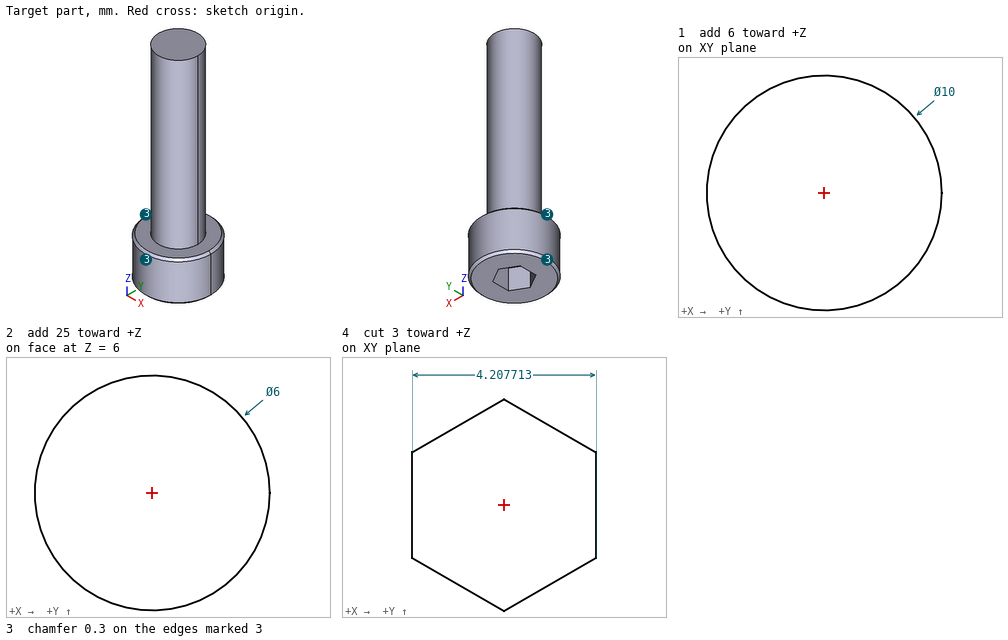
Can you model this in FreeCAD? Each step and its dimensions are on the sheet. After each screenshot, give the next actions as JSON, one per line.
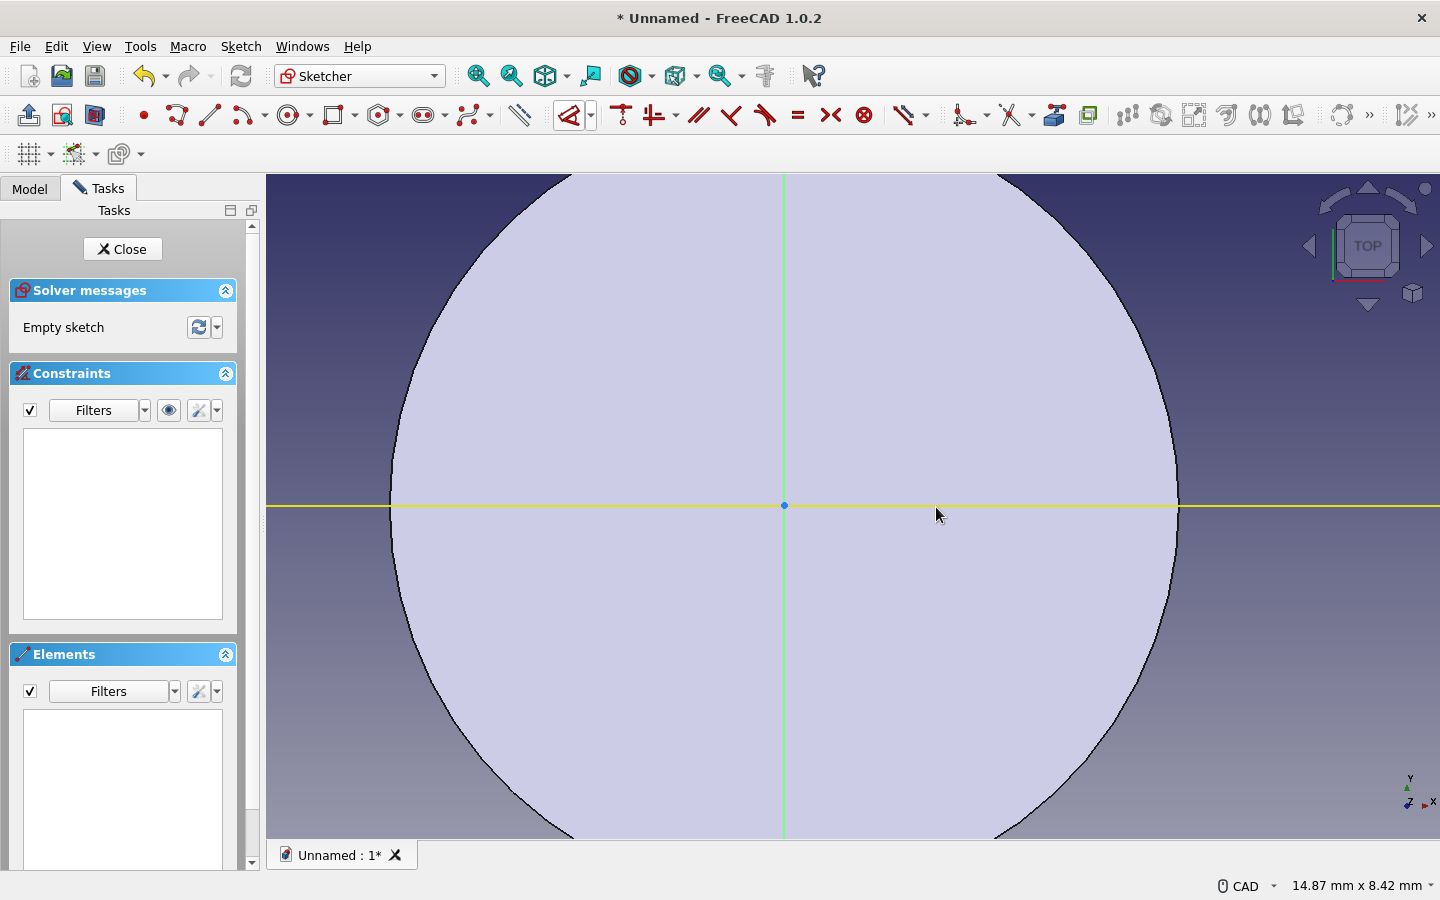
{"action": "left_click", "coordinate": [288, 116]}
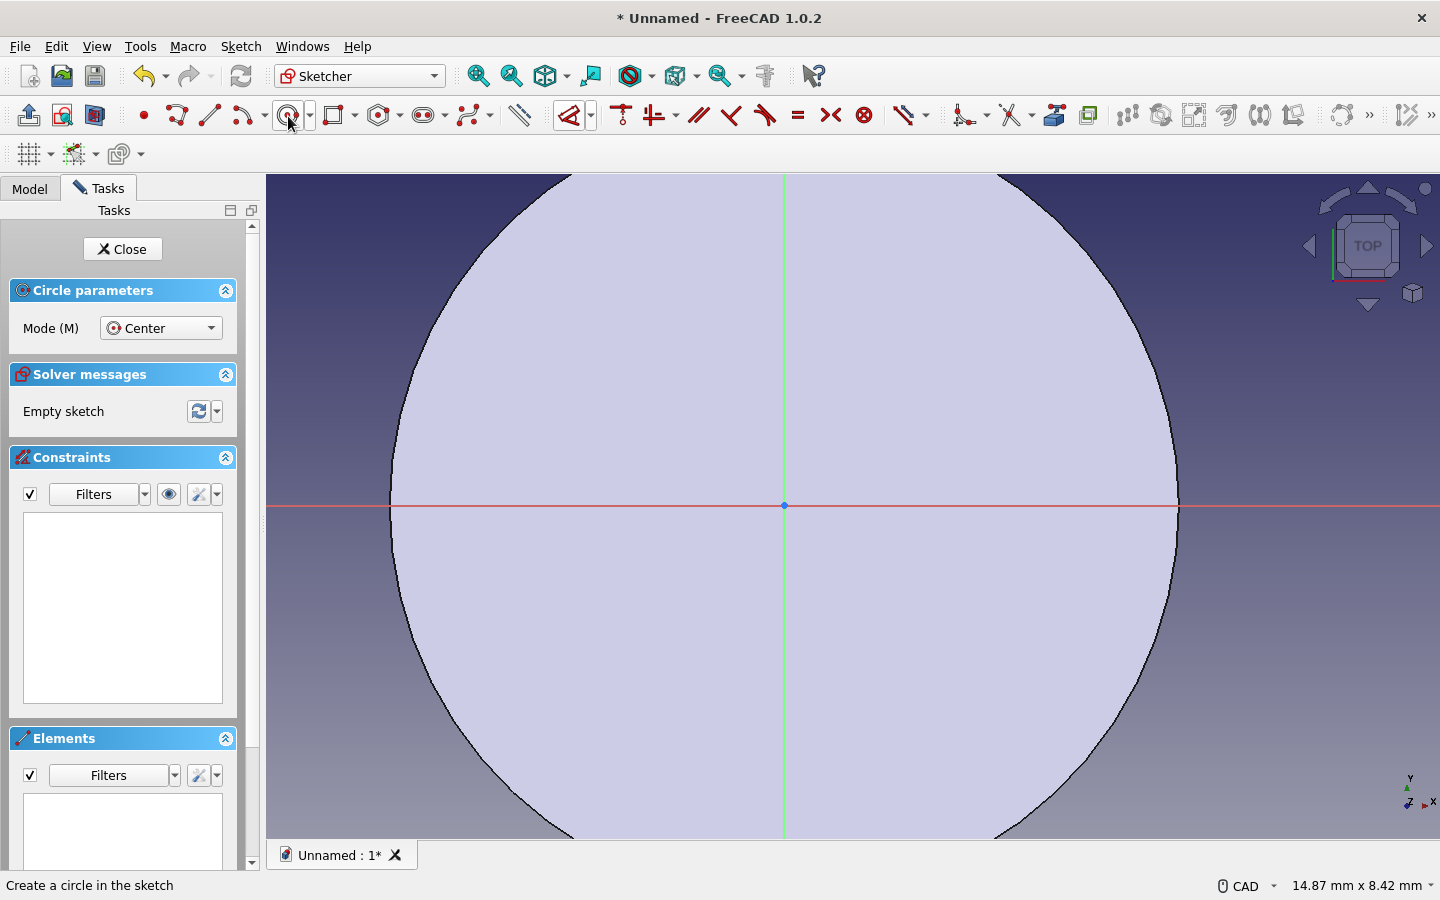
{"action": "left_click", "coordinate": [784, 506]}
{"action": "mouse_move", "coordinate": [952, 338]}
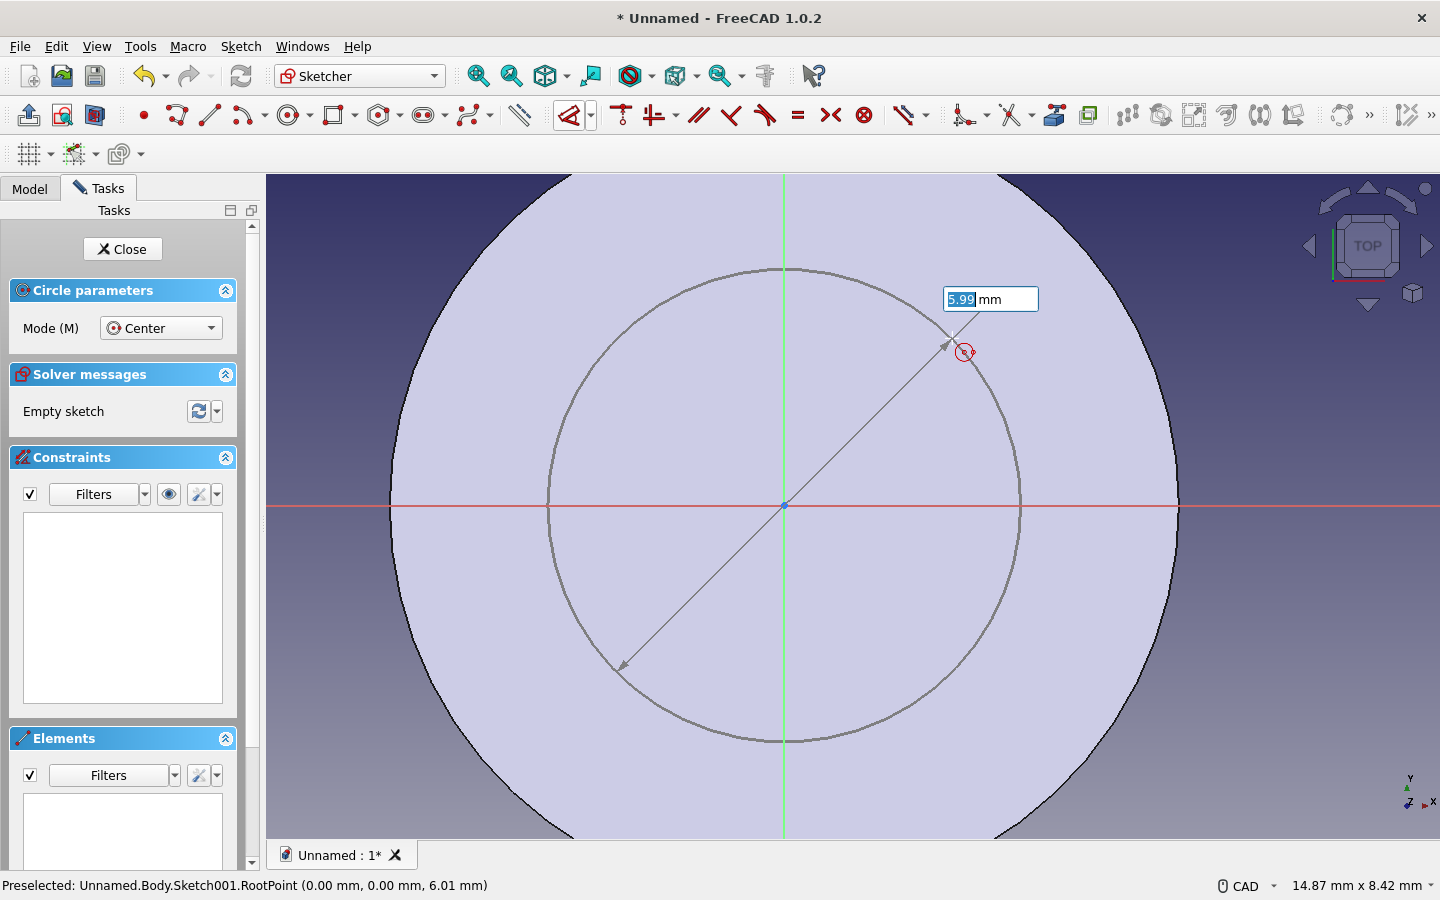
{"action": "type", "text": "6"}
{"action": "key", "text": "Return"}
{"action": "key", "text": "Escape"}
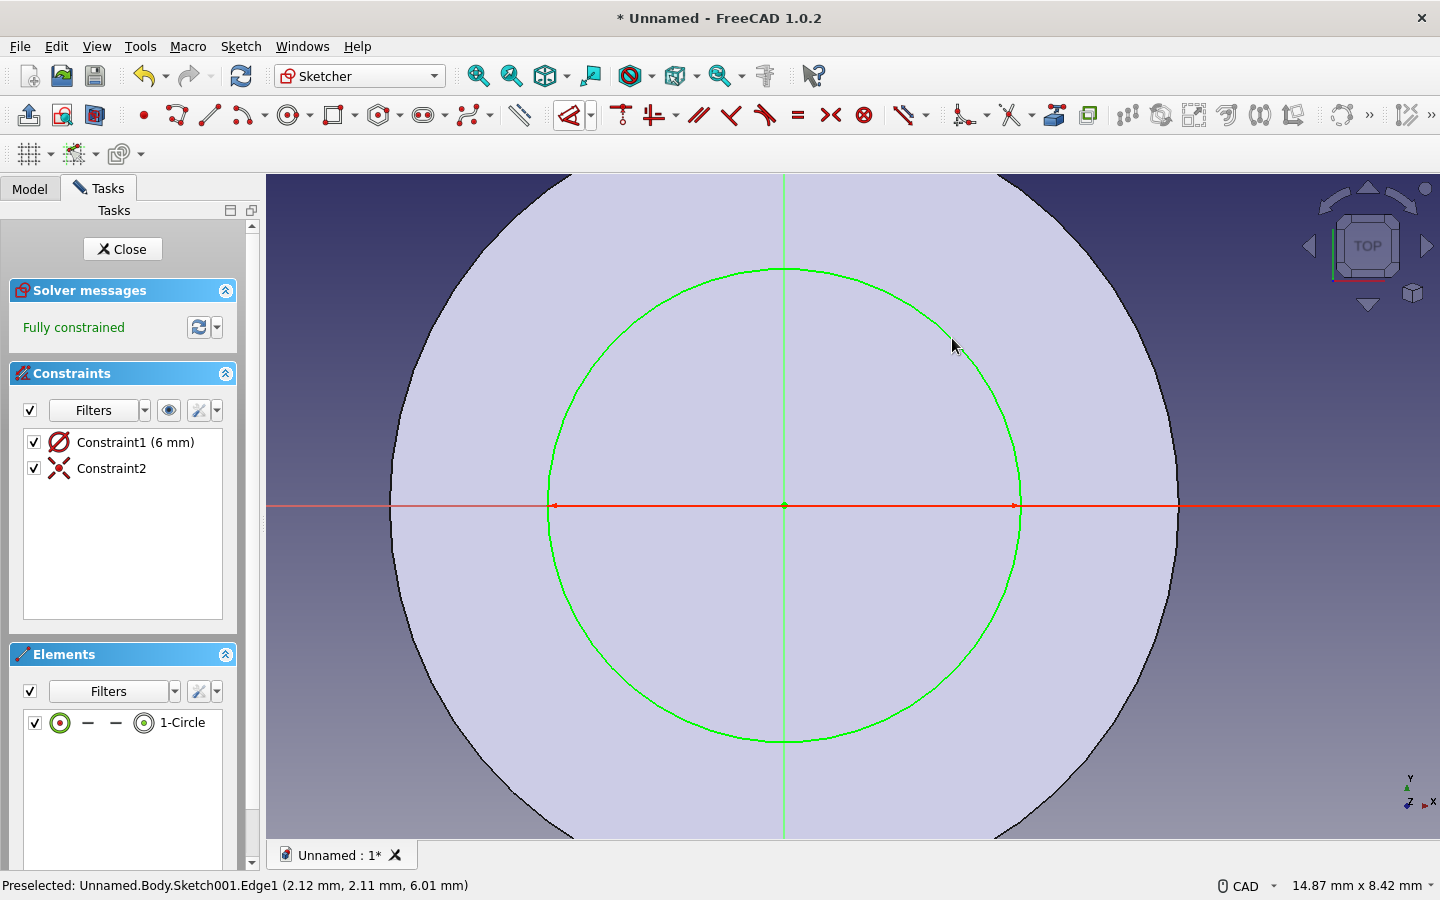
{"action": "left_click", "coordinate": [123, 249]}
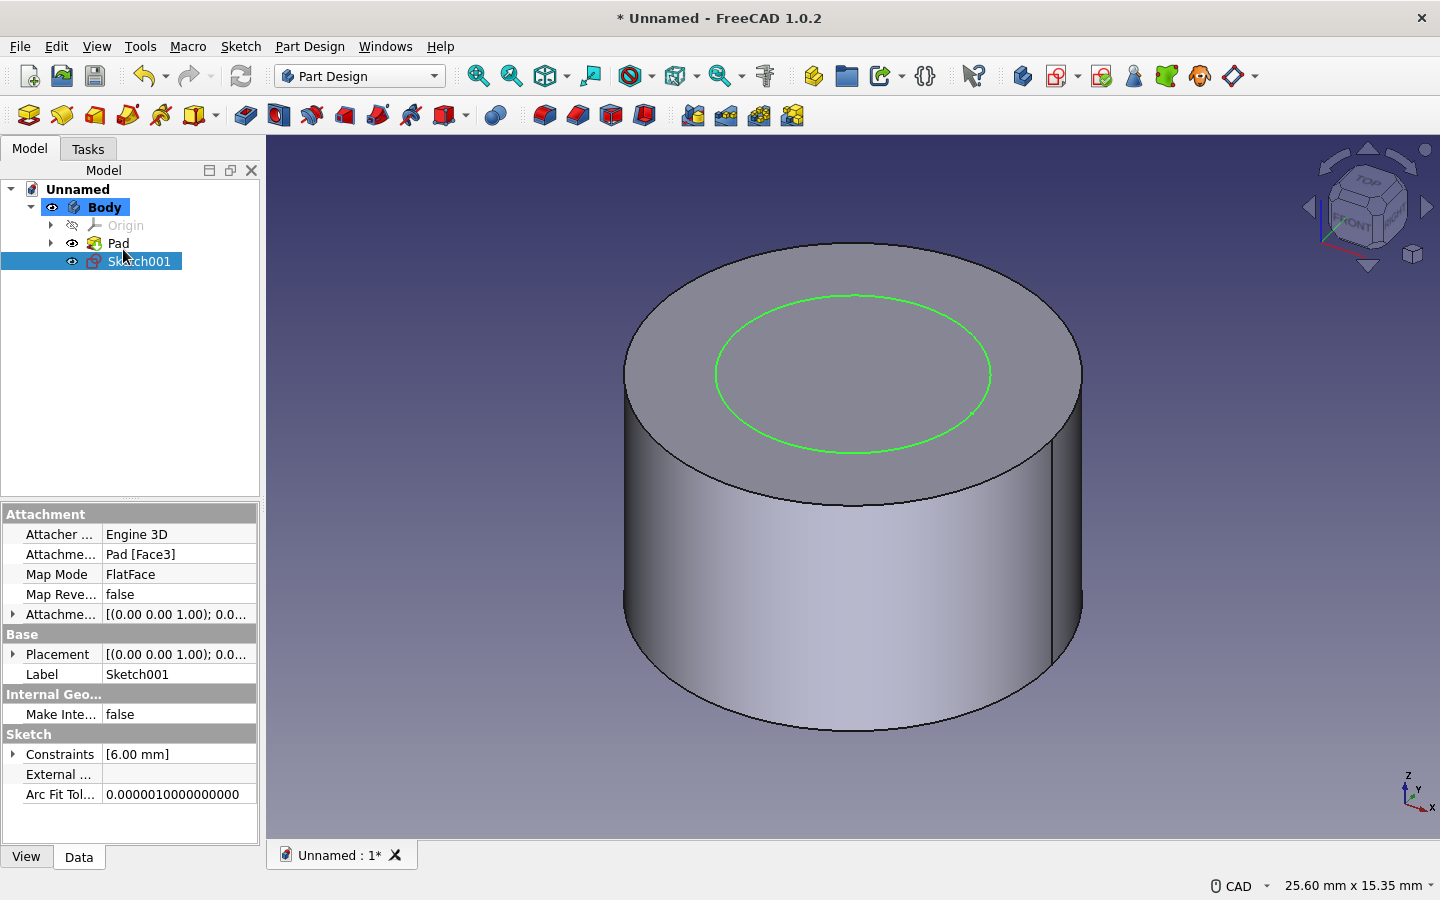
{"action": "left_click", "coordinate": [29, 116]}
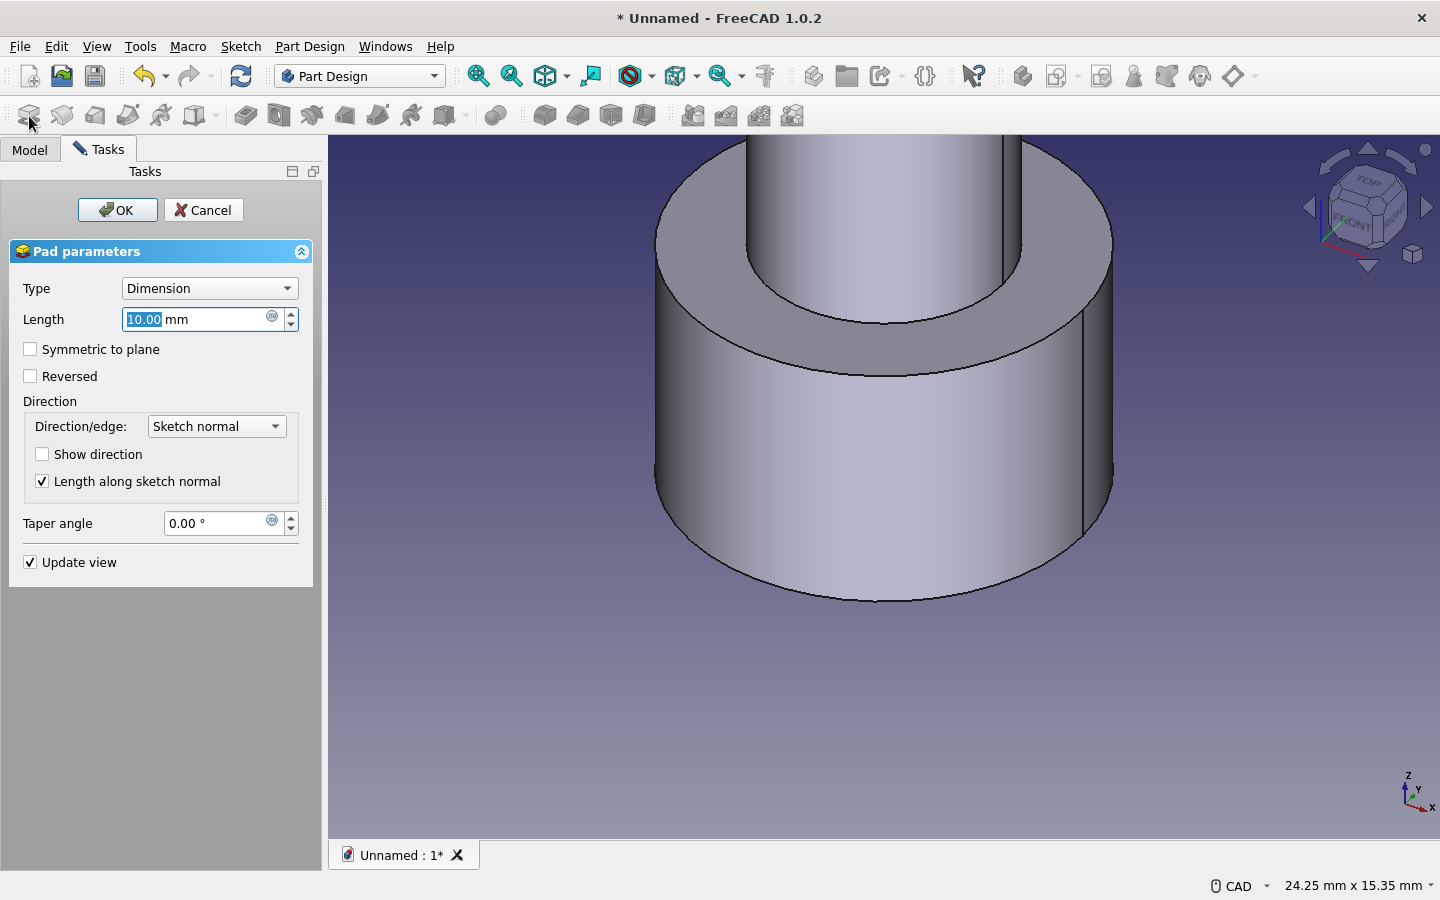
{"action": "type", "text": "25"}
{"action": "key", "text": "Tab"}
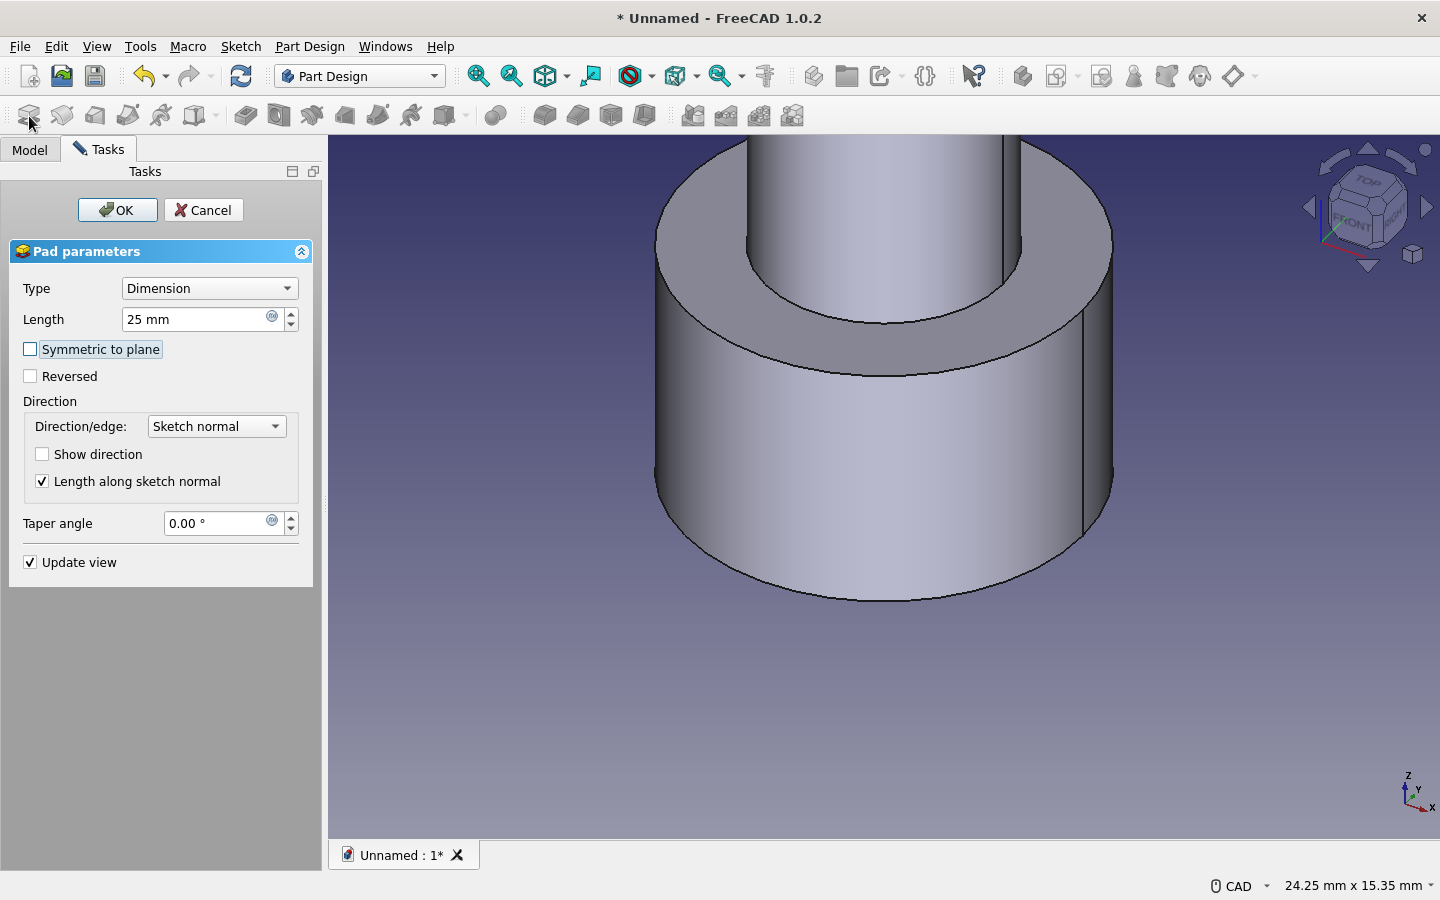
{"action": "left_click", "coordinate": [118, 210]}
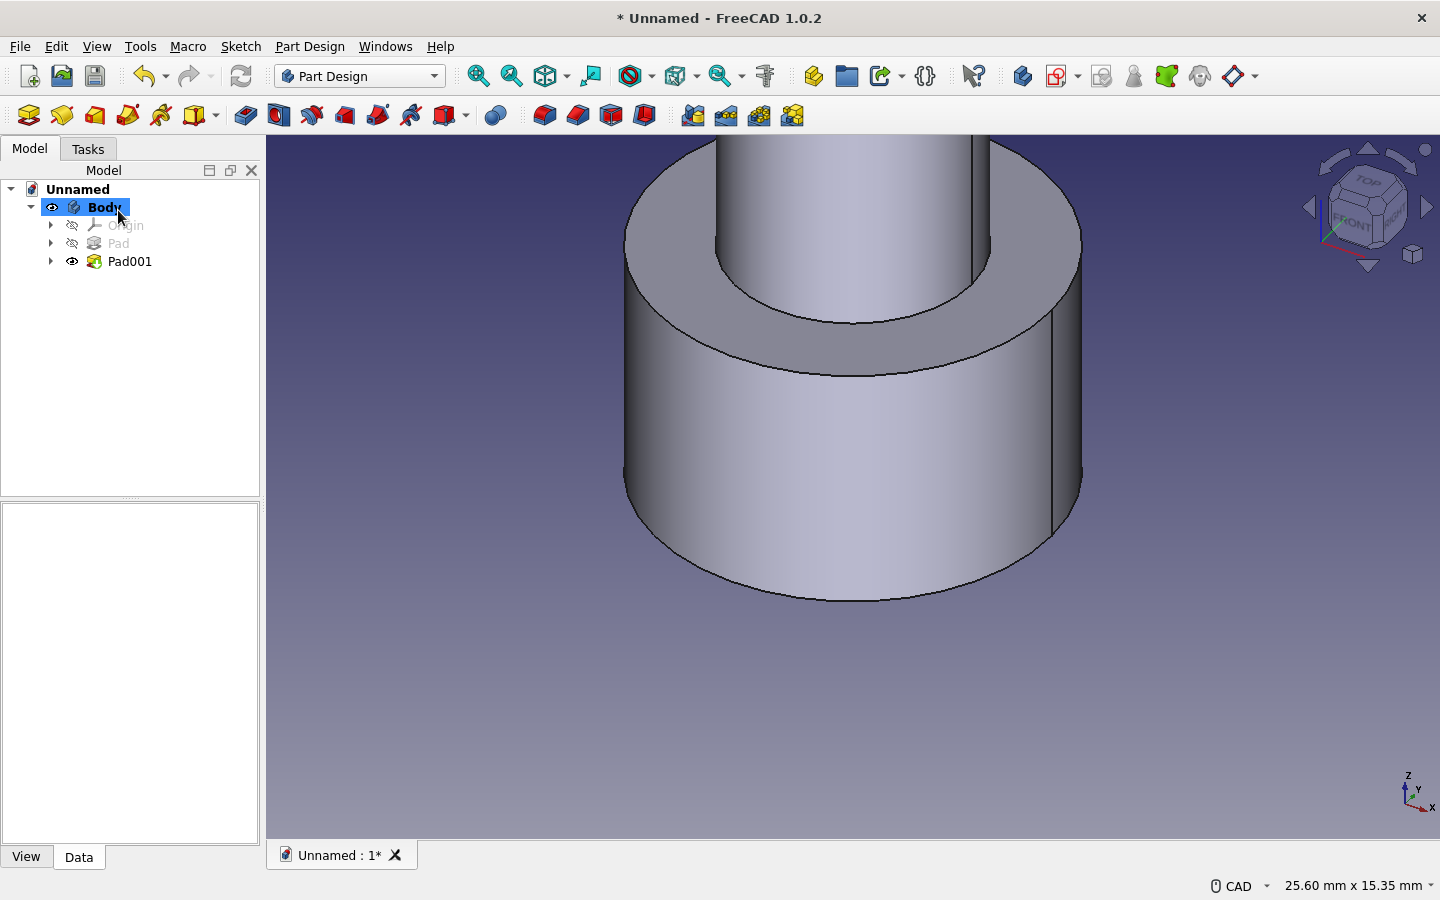
{"action": "left_click", "coordinate": [479, 76]}